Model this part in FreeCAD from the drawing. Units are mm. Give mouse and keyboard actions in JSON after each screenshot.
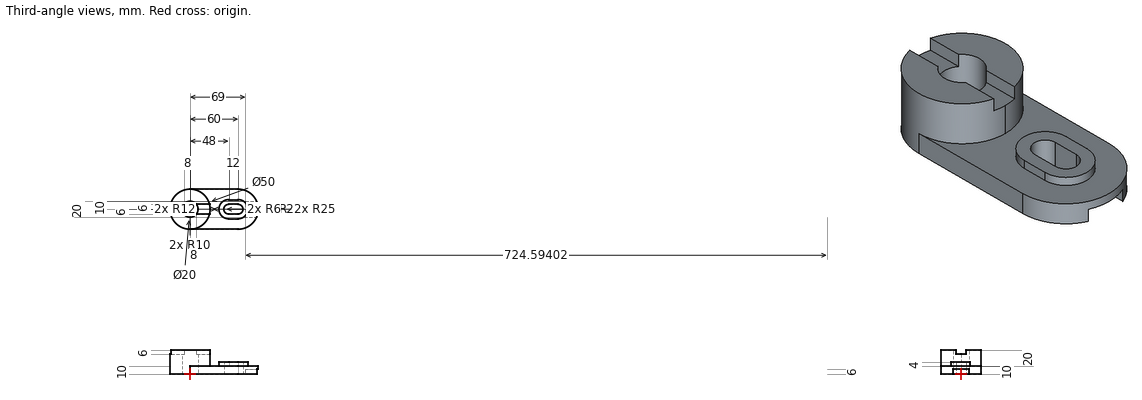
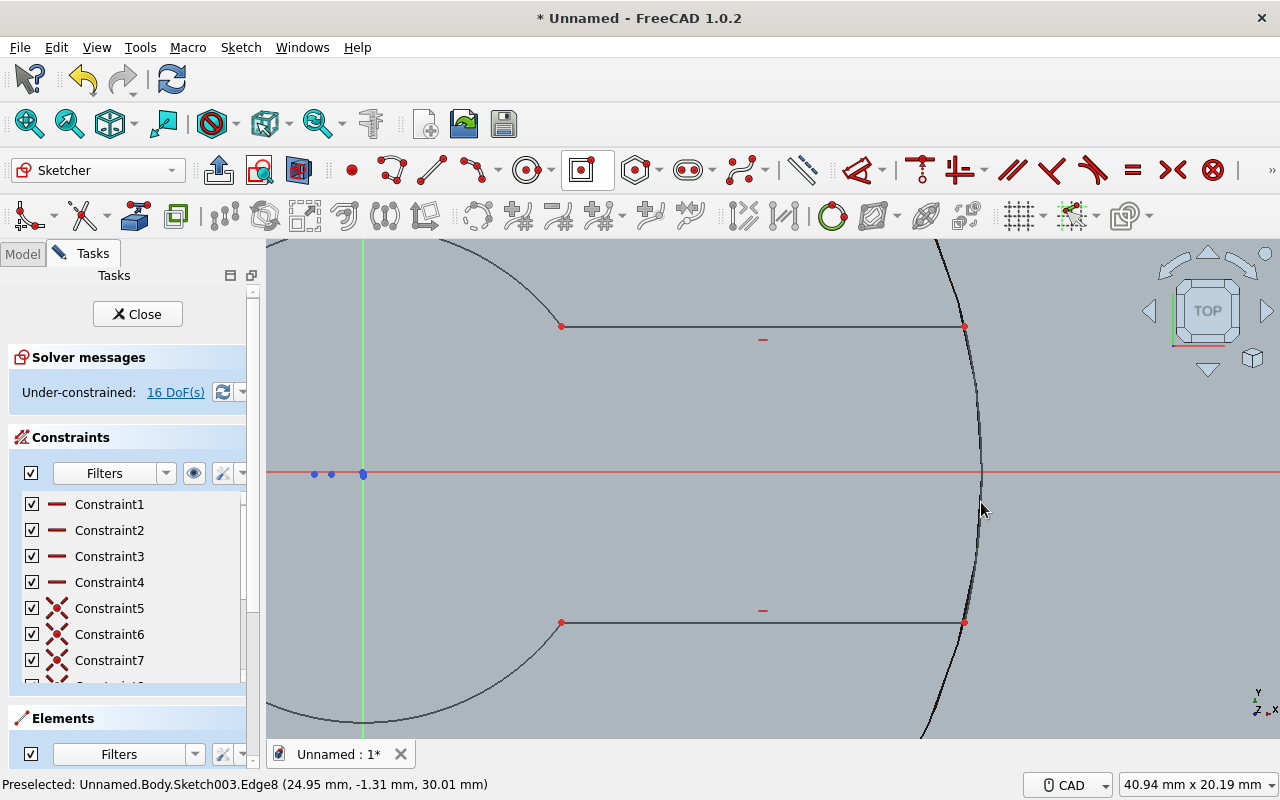
{"action": "scroll", "coordinate": [983, 503], "scroll_direction": "down", "scroll_amount": 4}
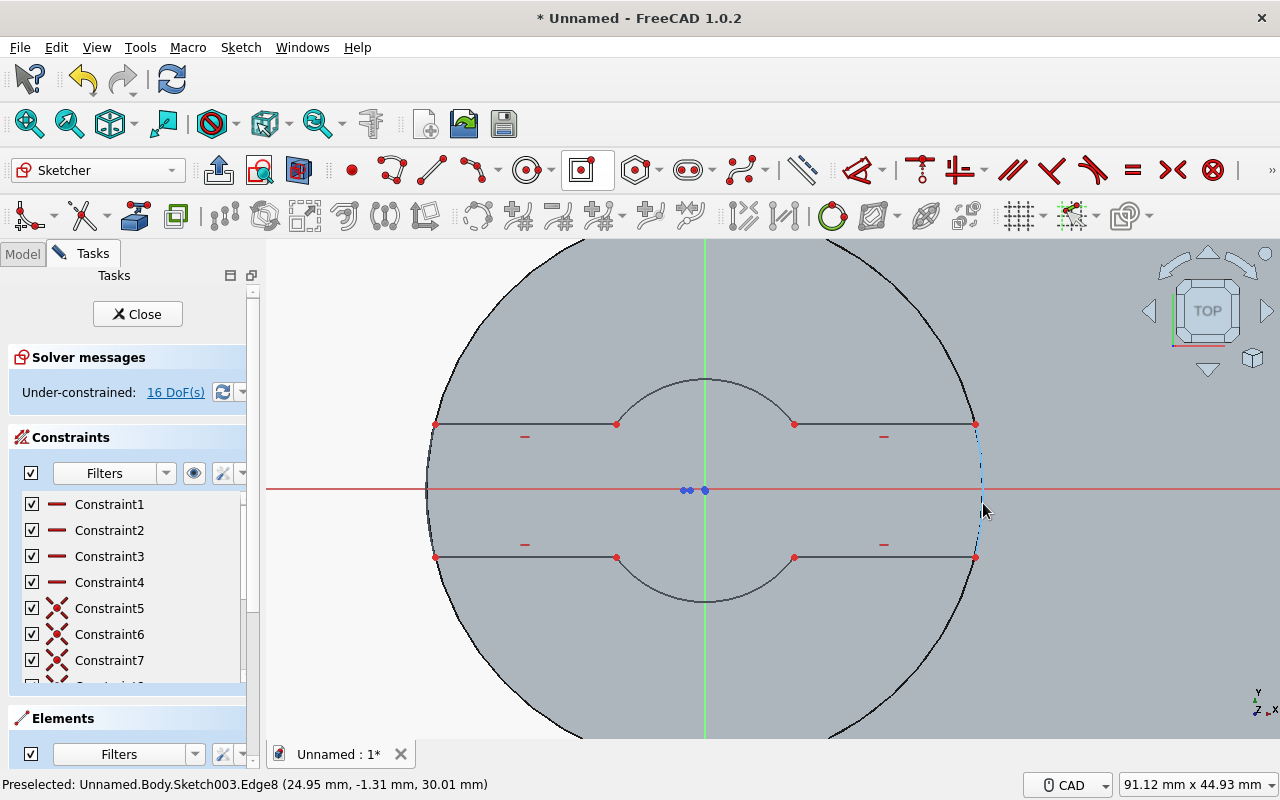
{"action": "left_click", "coordinate": [745, 387]}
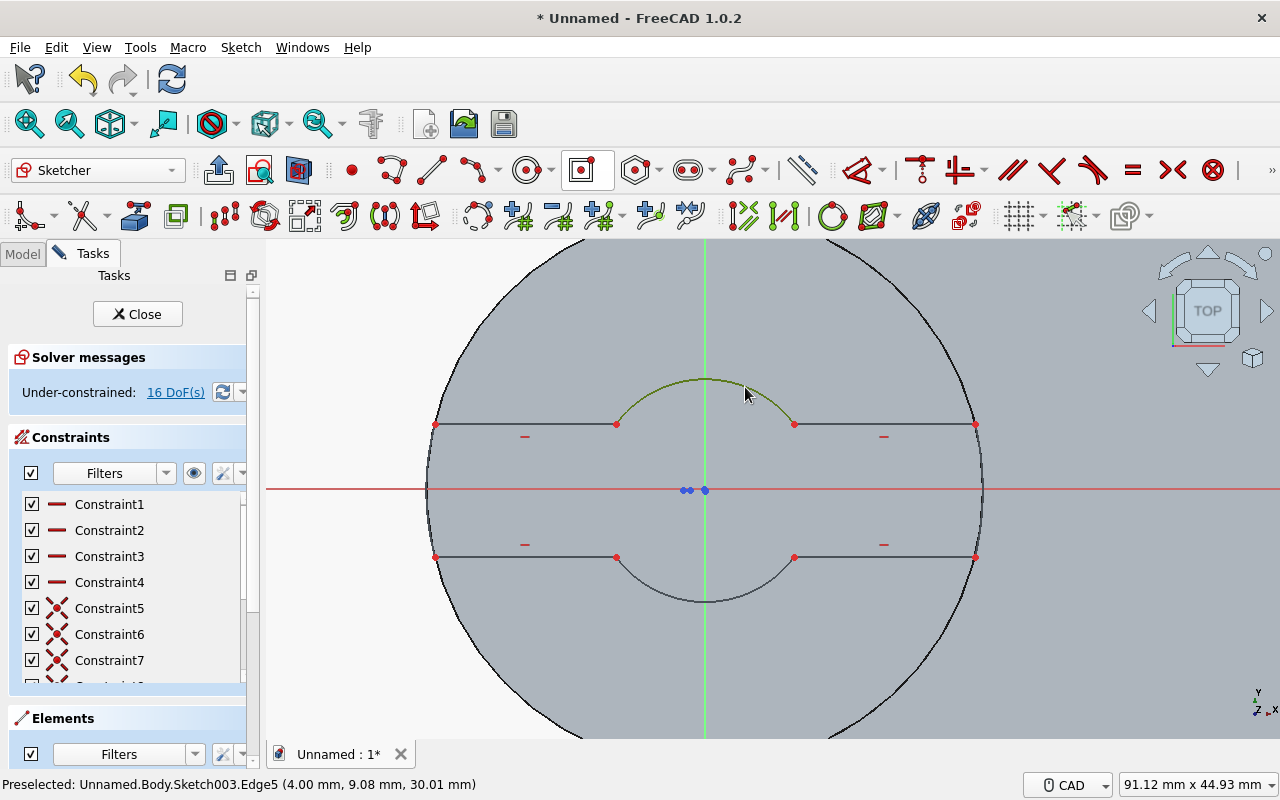
{"action": "left_click", "coordinate": [428, 464]}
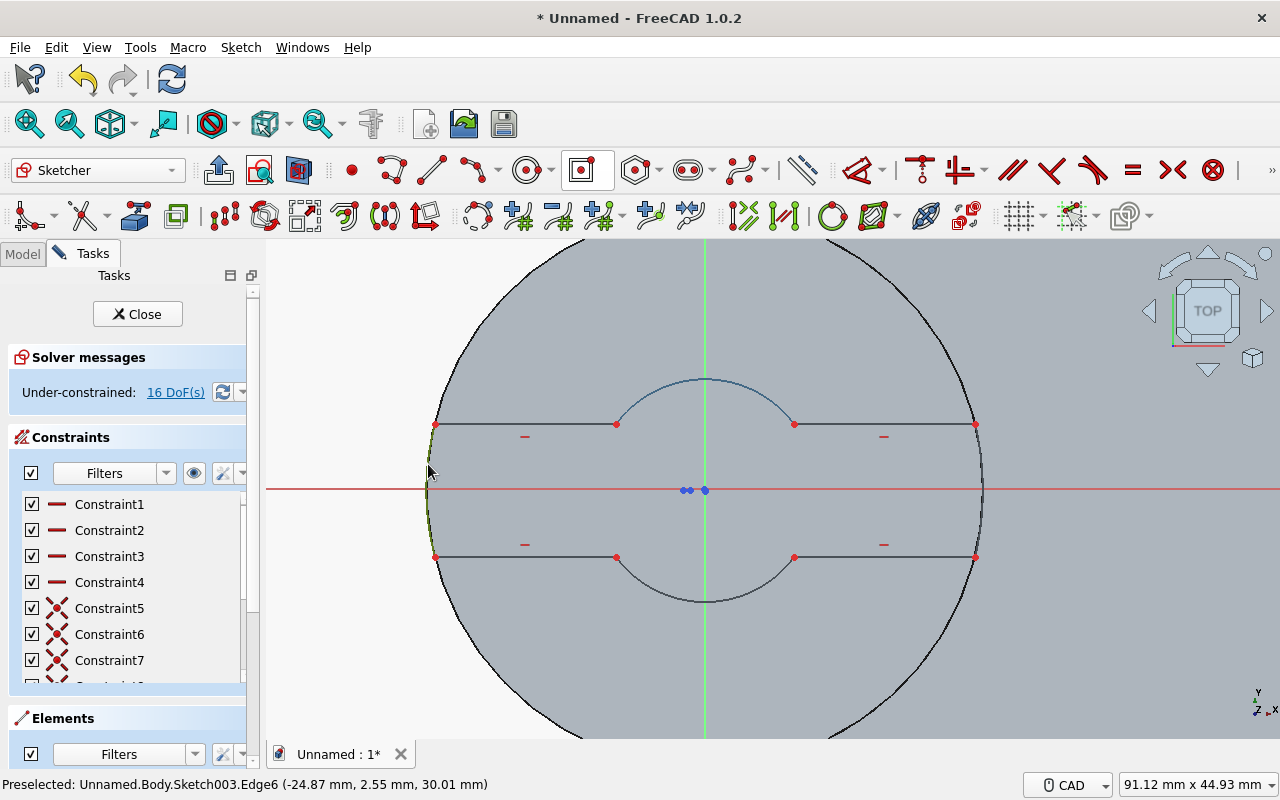
{"action": "left_click", "coordinate": [920, 170]}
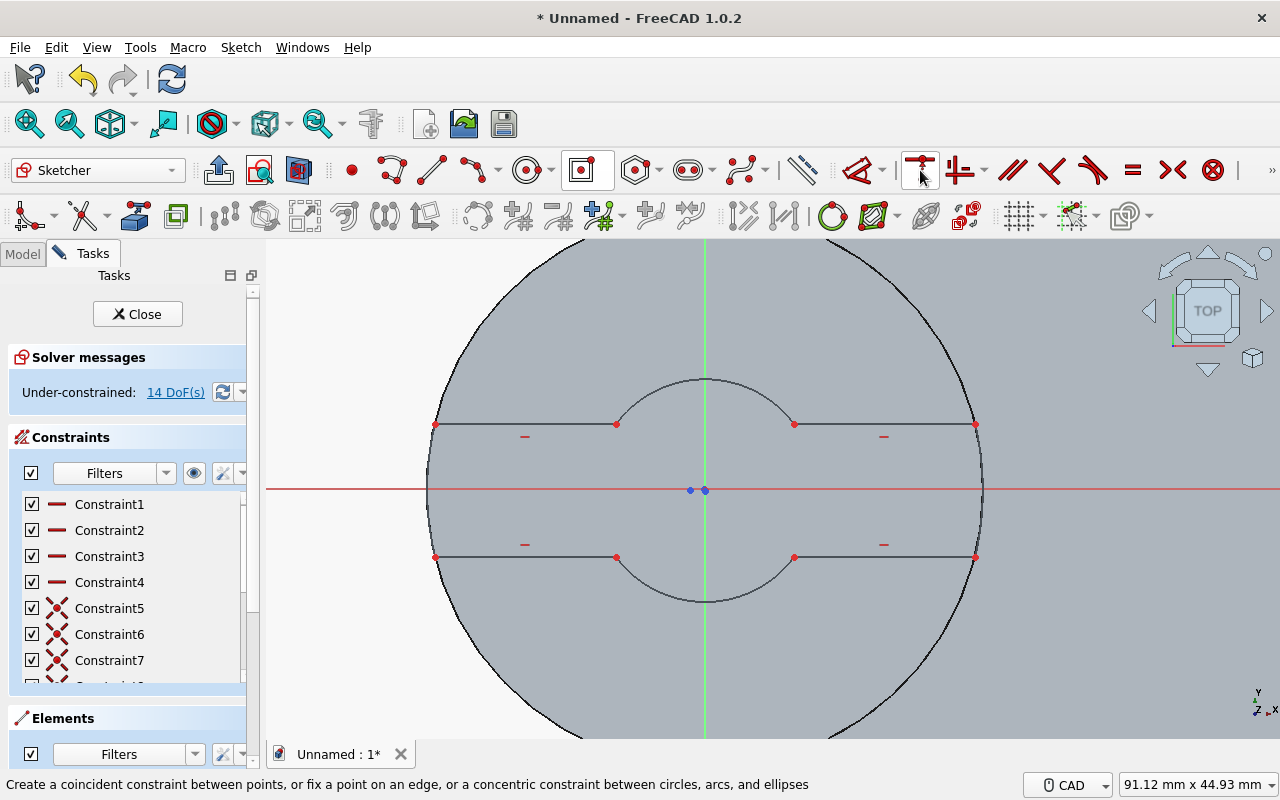
{"action": "left_click", "coordinate": [745, 387]}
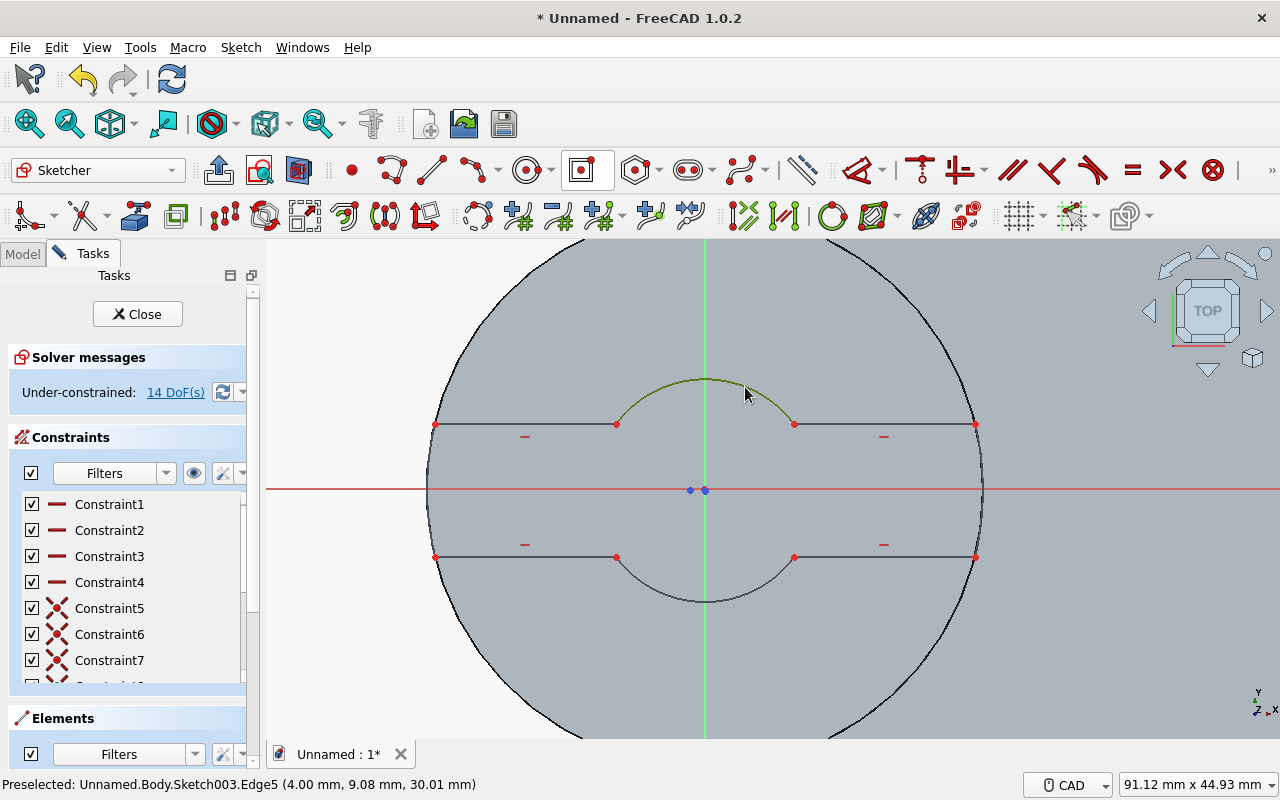
{"action": "left_click", "coordinate": [665, 594]}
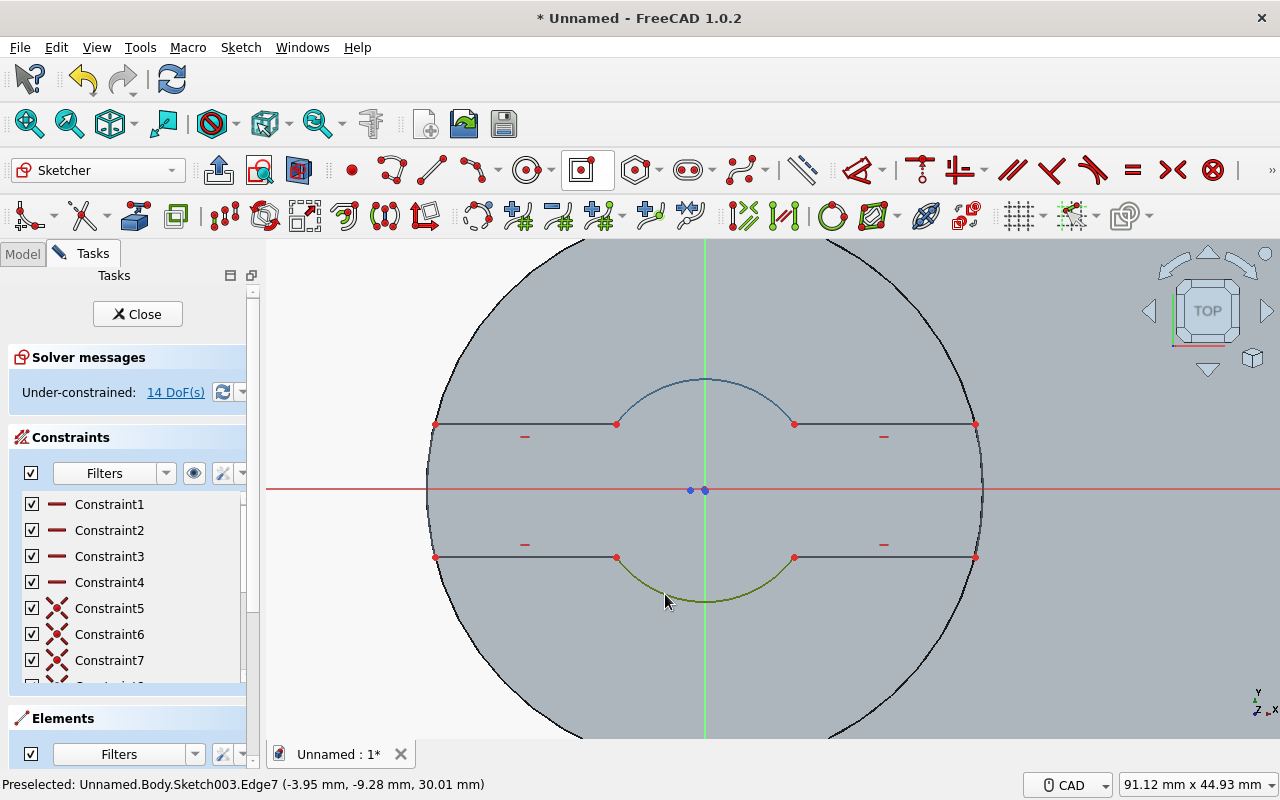
{"action": "left_click", "coordinate": [920, 170]}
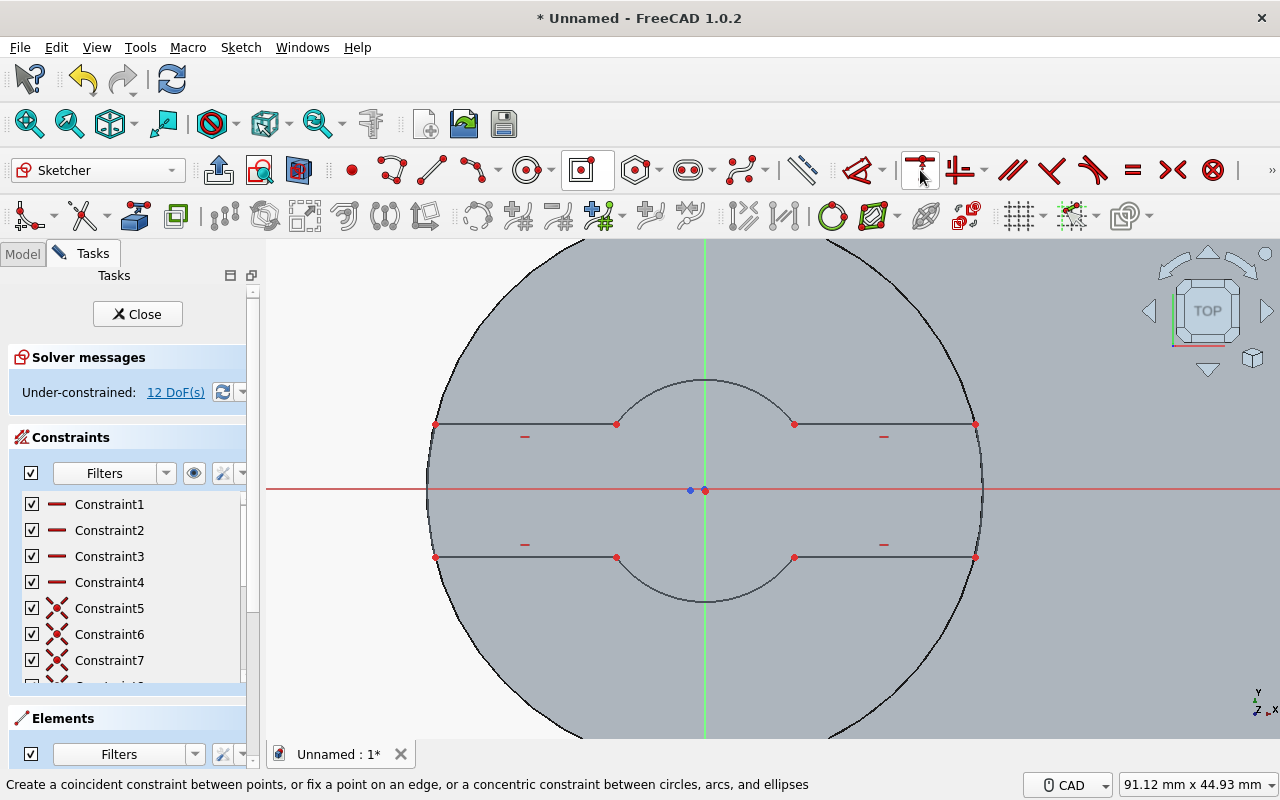
{"action": "left_click", "coordinate": [745, 387]}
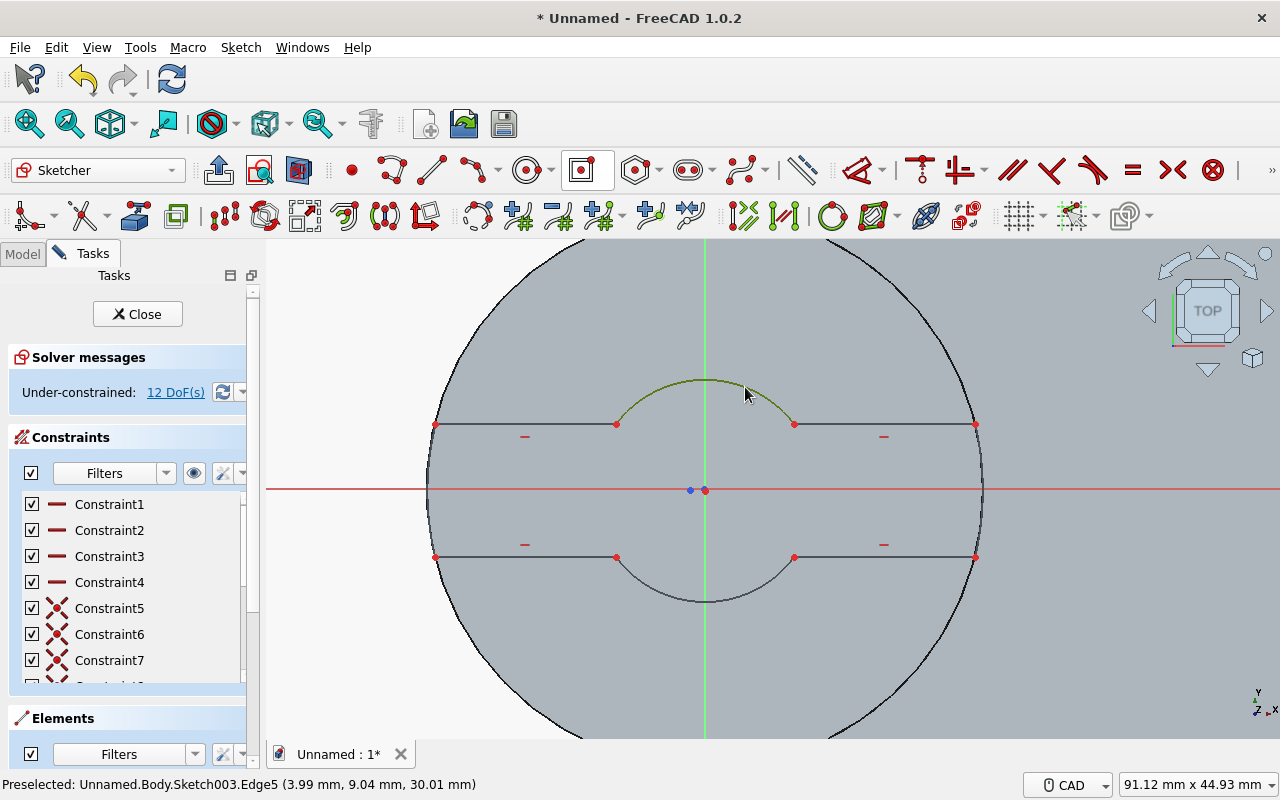
{"action": "left_click", "coordinate": [982, 517]}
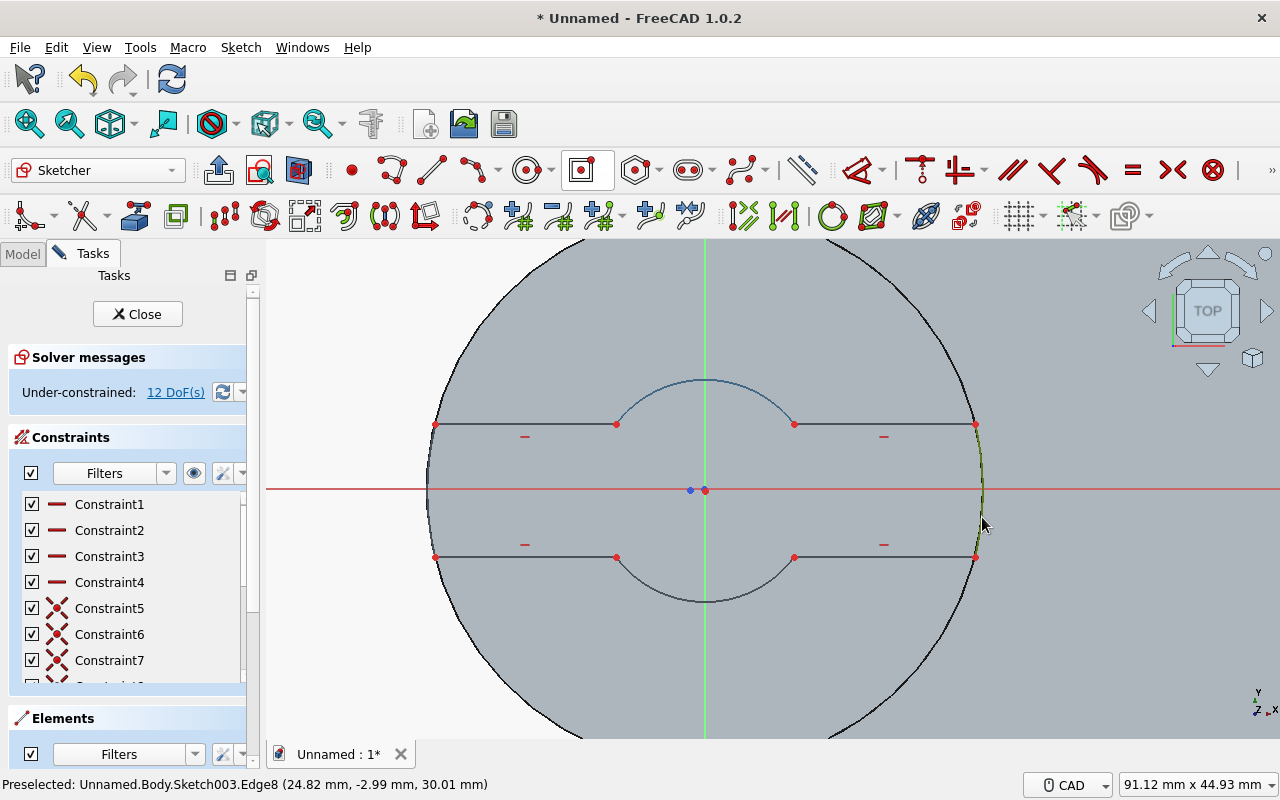
{"action": "left_click", "coordinate": [920, 170]}